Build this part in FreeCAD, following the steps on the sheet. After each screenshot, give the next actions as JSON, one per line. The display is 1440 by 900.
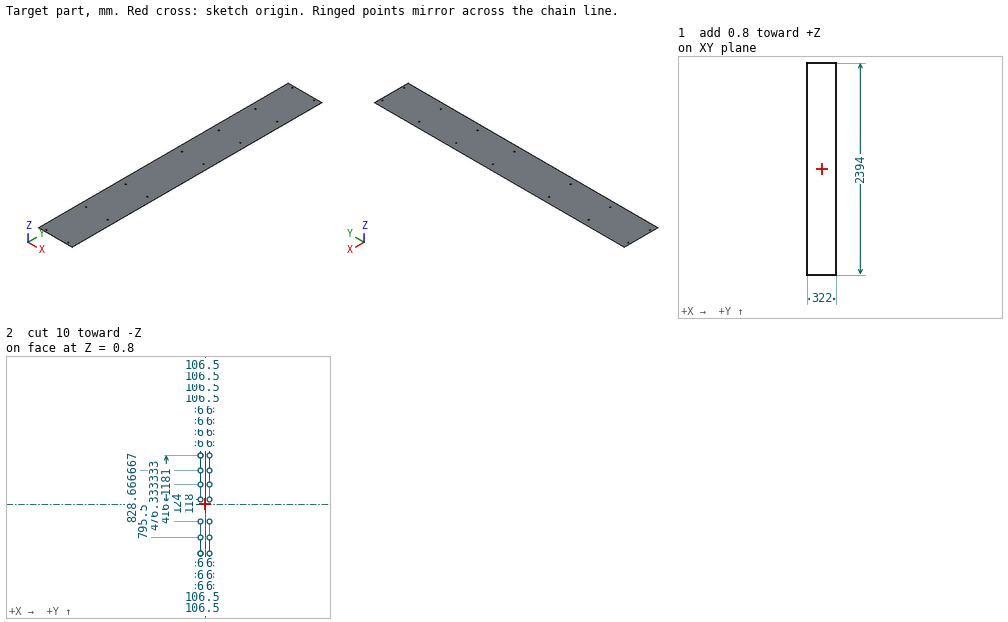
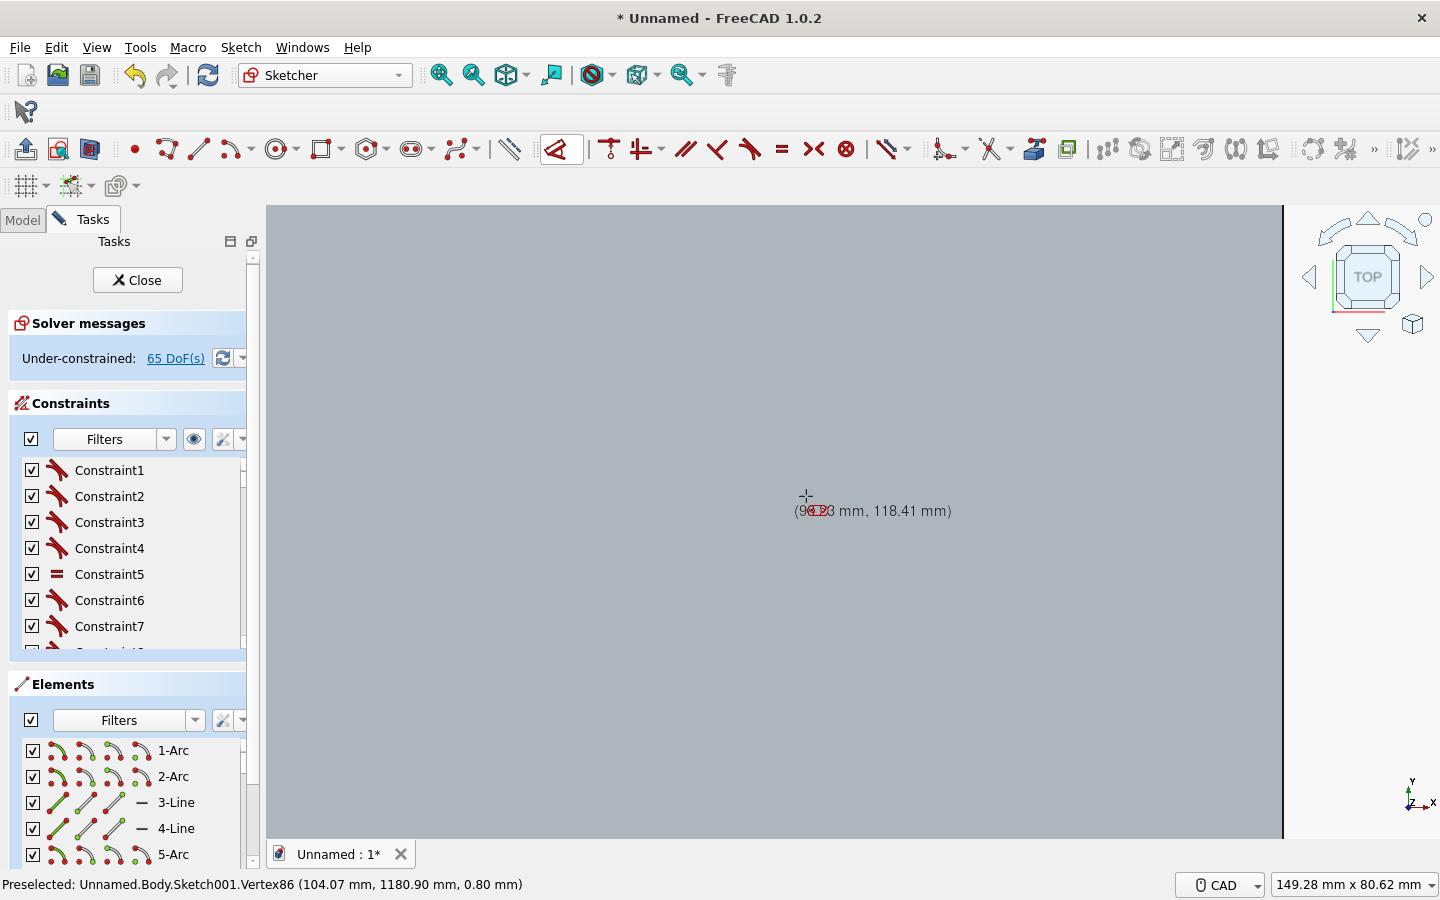
{"action": "scroll", "coordinate": [806, 496], "scroll_direction": "down", "scroll_amount": 18}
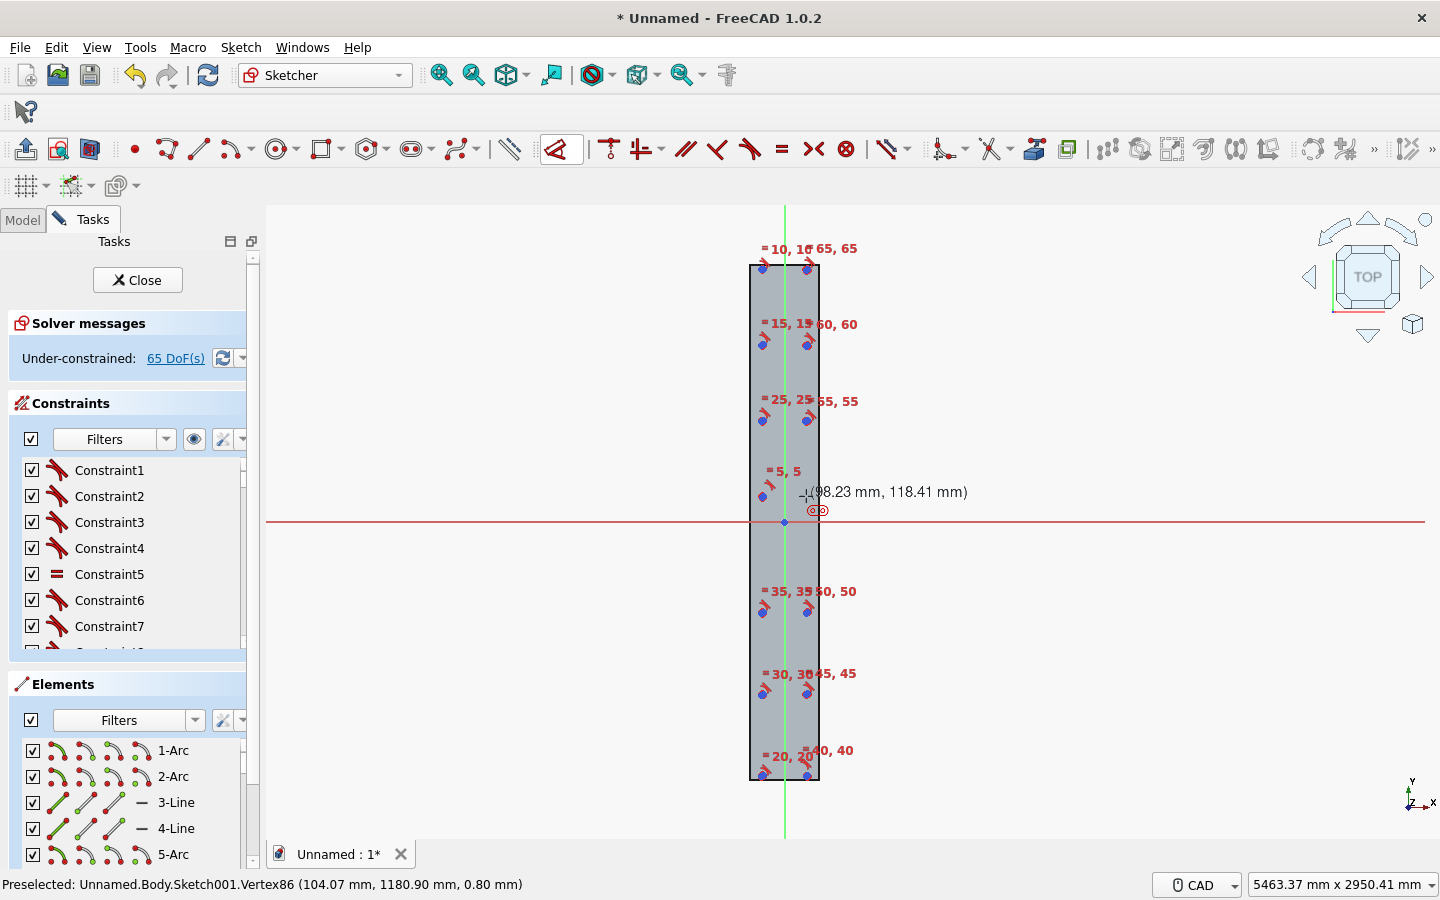
{"action": "left_click", "coordinate": [806, 496]}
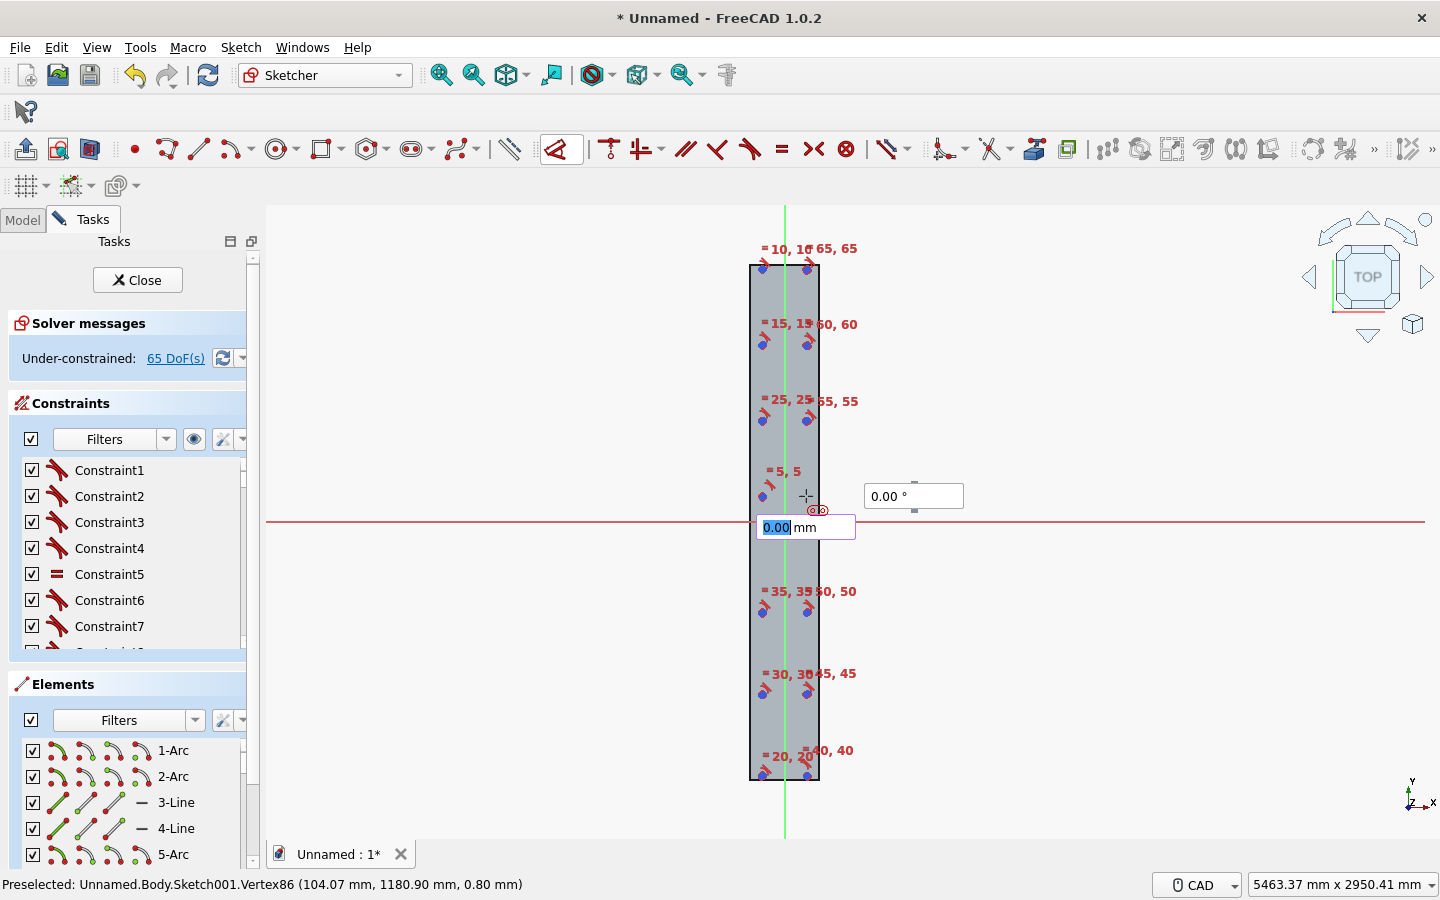
{"action": "scroll", "coordinate": [808, 496], "scroll_direction": "up", "scroll_amount": 13}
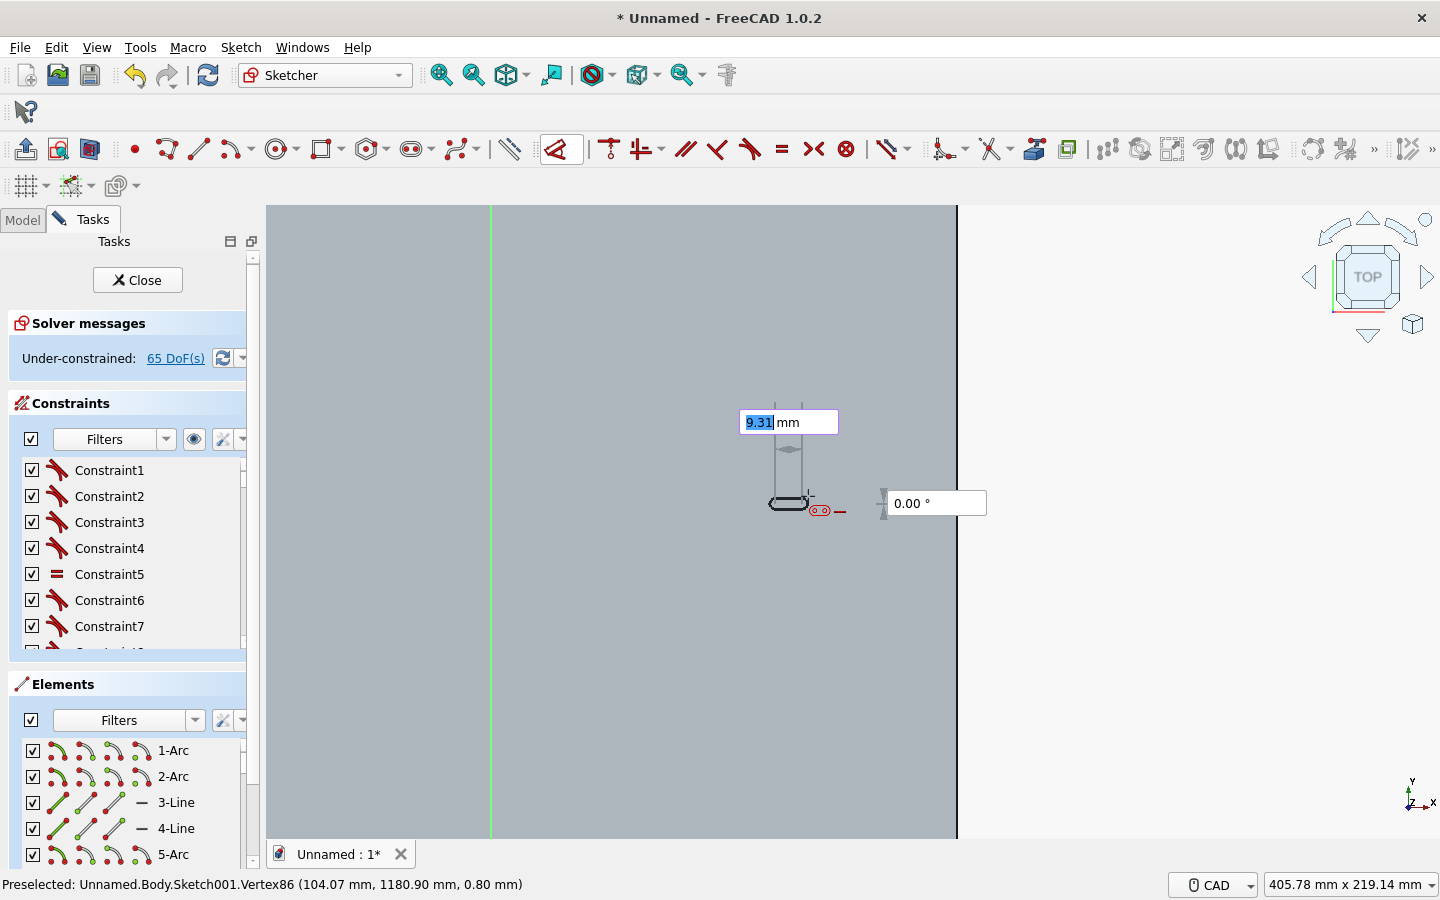
{"action": "left_click", "coordinate": [799, 490]}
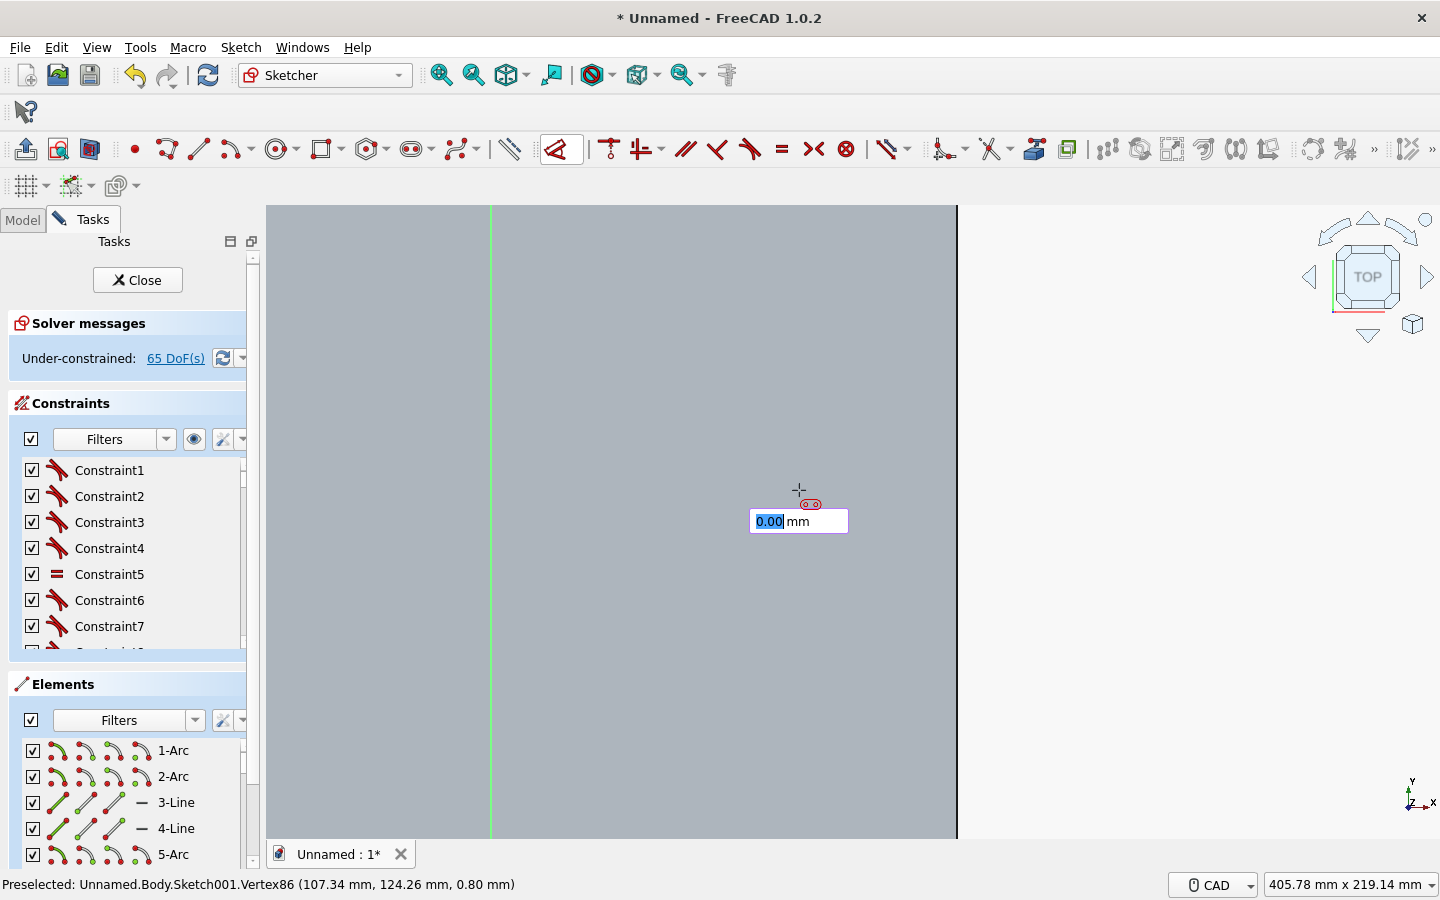
{"action": "scroll", "coordinate": [791, 488], "scroll_direction": "up", "scroll_amount": 4}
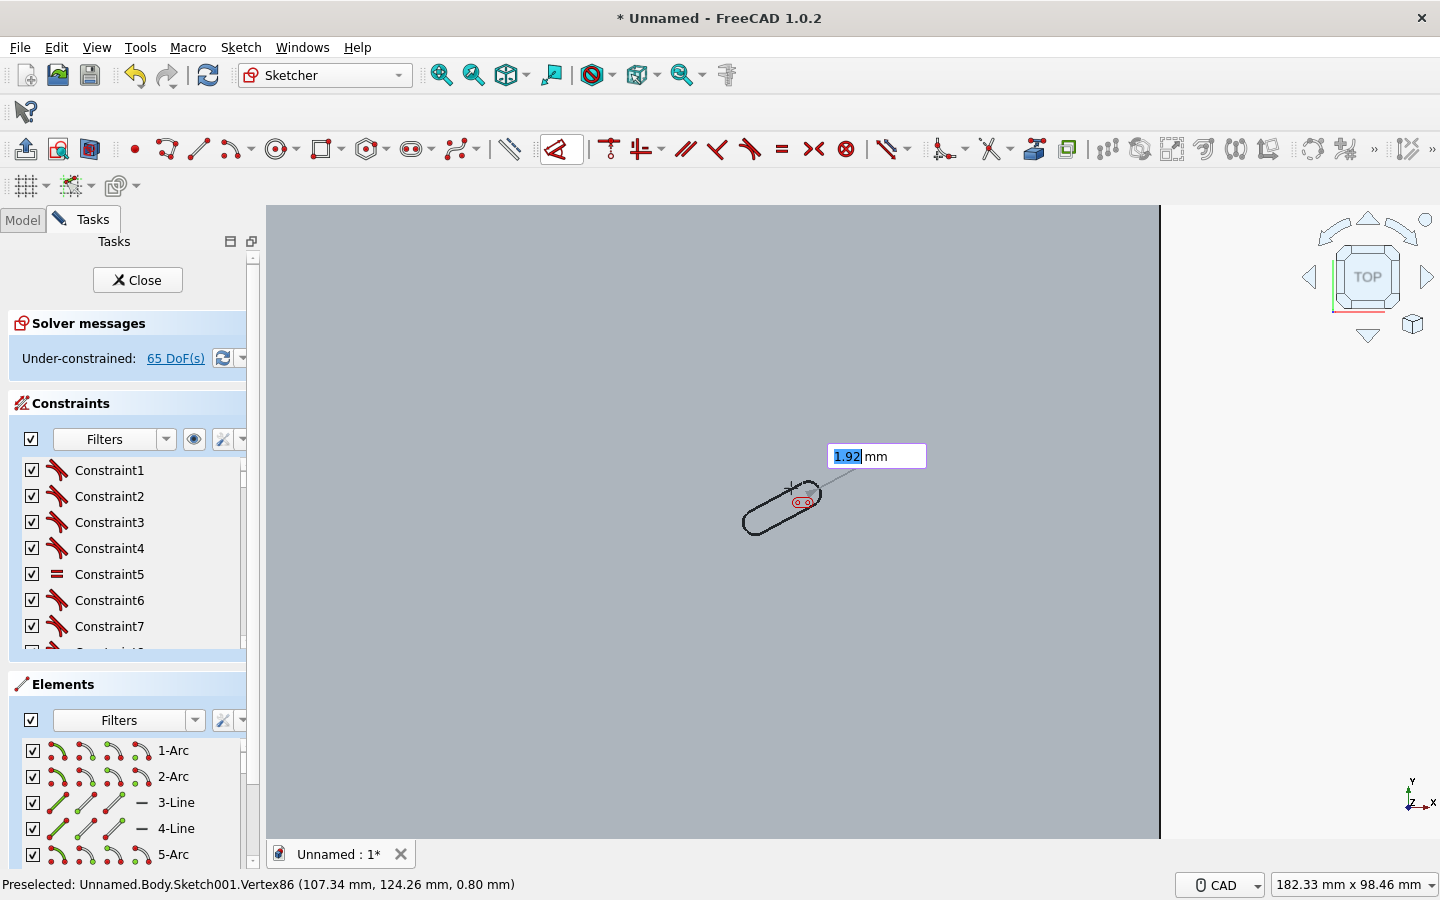
{"action": "left_click", "coordinate": [789, 486]}
{"action": "key", "text": "Escape"}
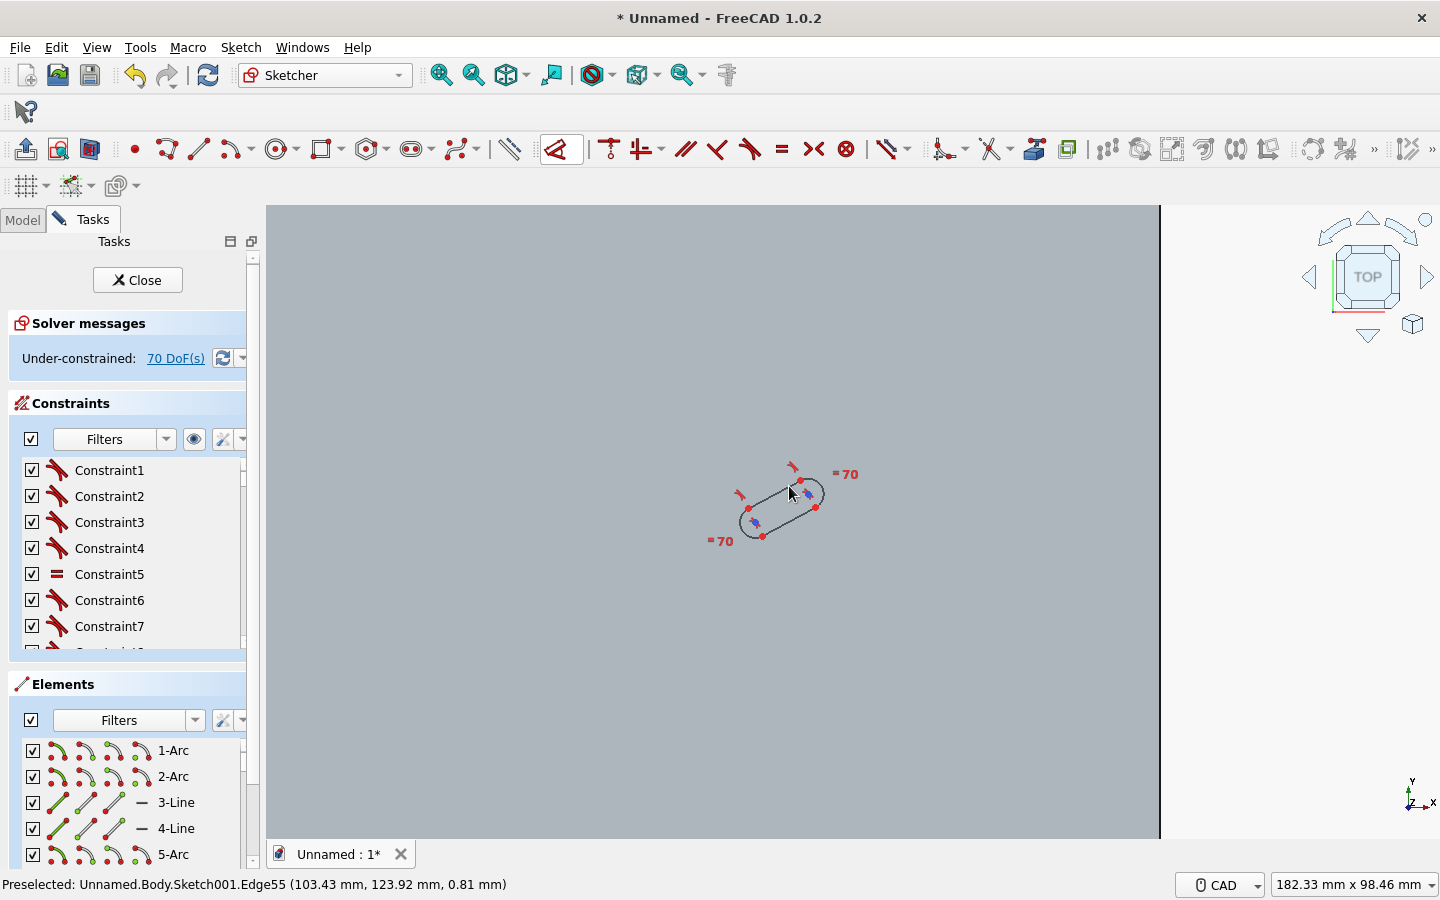
{"action": "scroll", "coordinate": [807, 496], "scroll_direction": "down", "scroll_amount": 17}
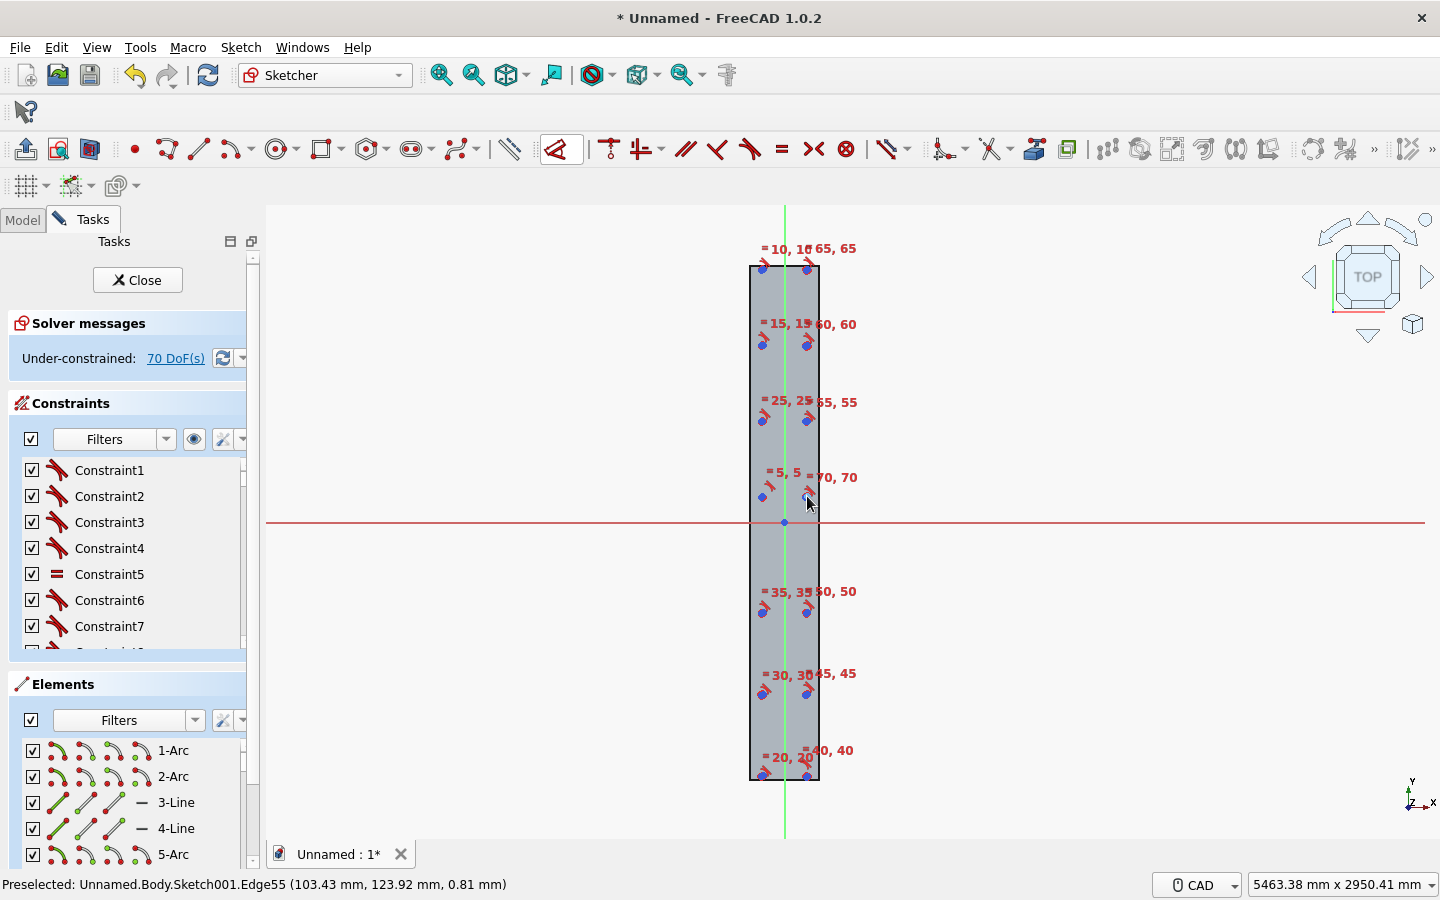
{"action": "scroll", "coordinate": [762, 497], "scroll_direction": "up", "scroll_amount": 13}